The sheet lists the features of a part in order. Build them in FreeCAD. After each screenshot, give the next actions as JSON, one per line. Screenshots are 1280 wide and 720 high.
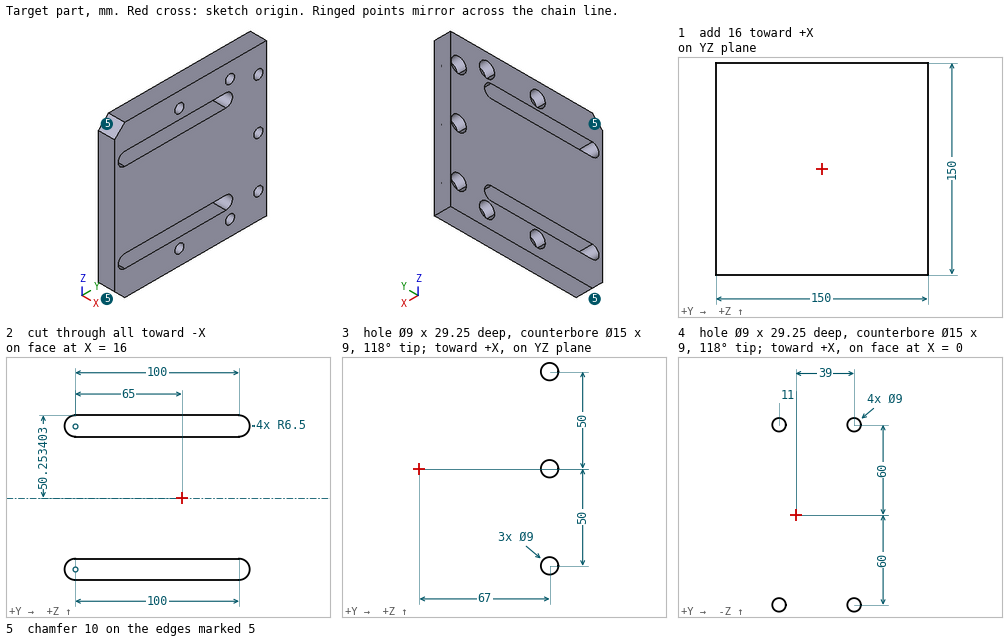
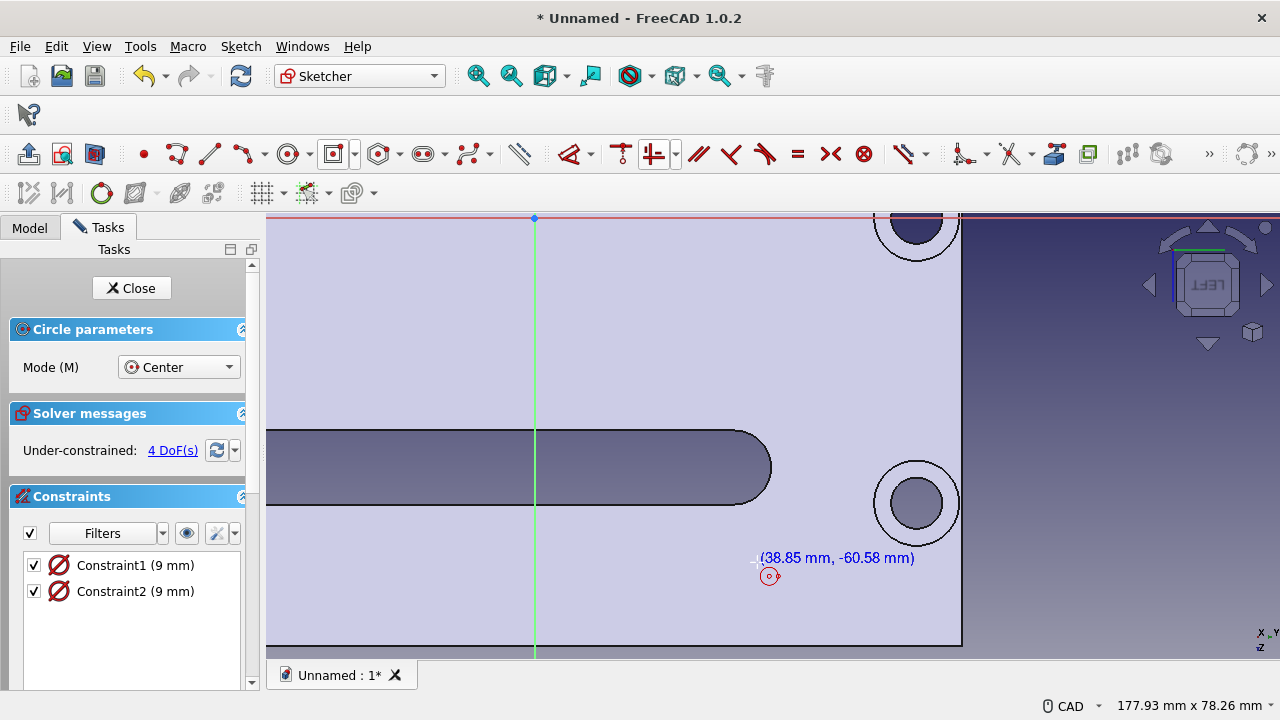
{"action": "left_click", "coordinate": [757, 560]}
{"action": "mouse_move", "coordinate": [775, 542]}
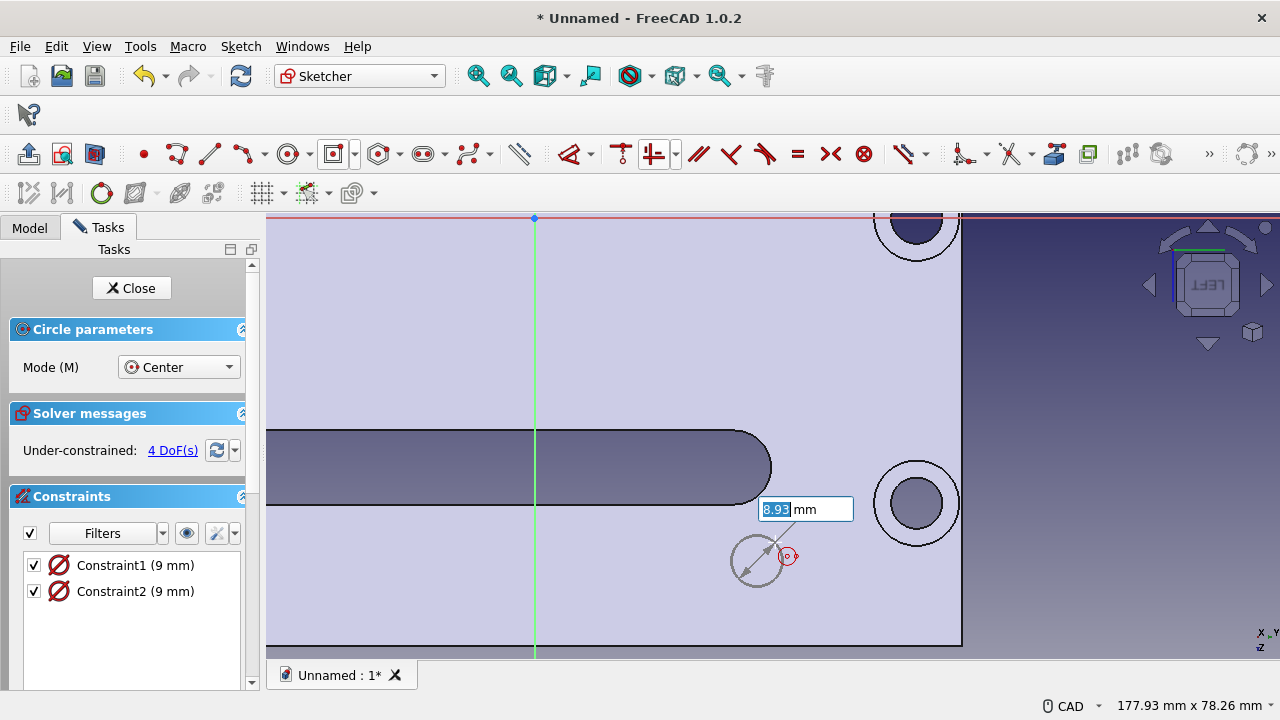
{"action": "type", "text": "9"}
{"action": "key", "text": "Return"}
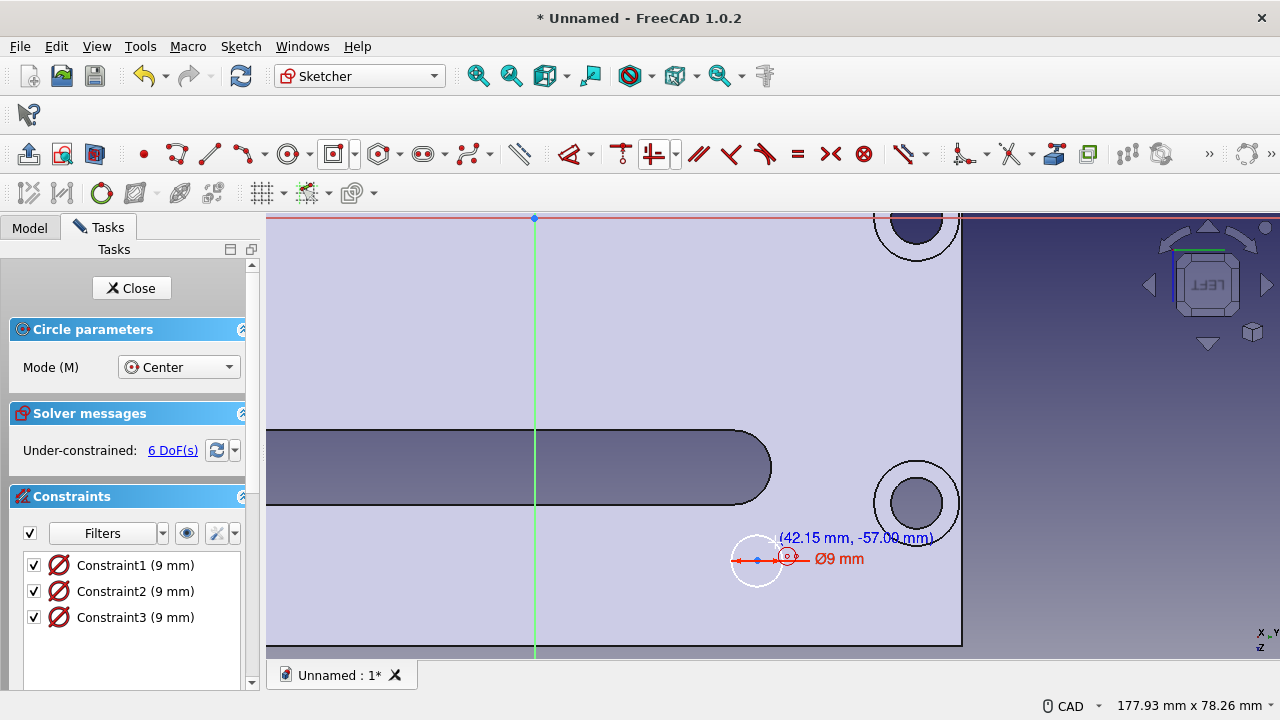
{"action": "left_click", "coordinate": [472, 560]}
{"action": "mouse_move", "coordinate": [490, 542]}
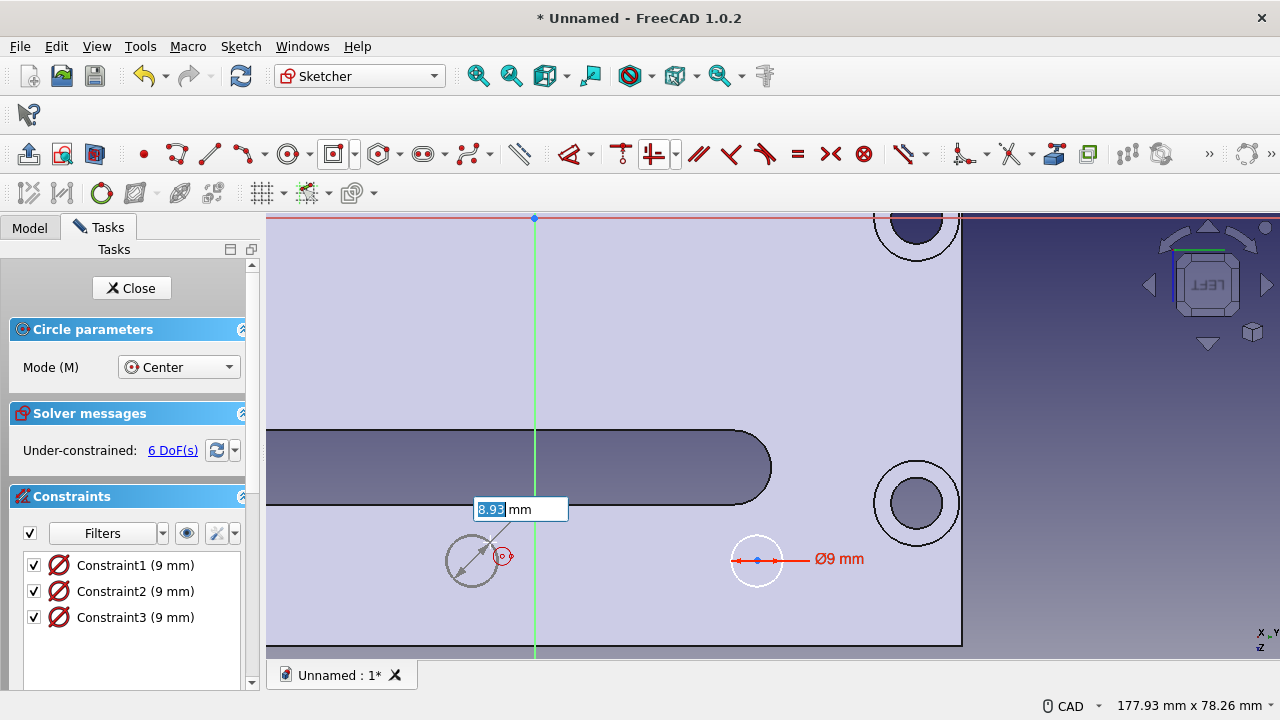
{"action": "type", "text": "9"}
{"action": "key", "text": "Return"}
{"action": "key", "text": "Escape"}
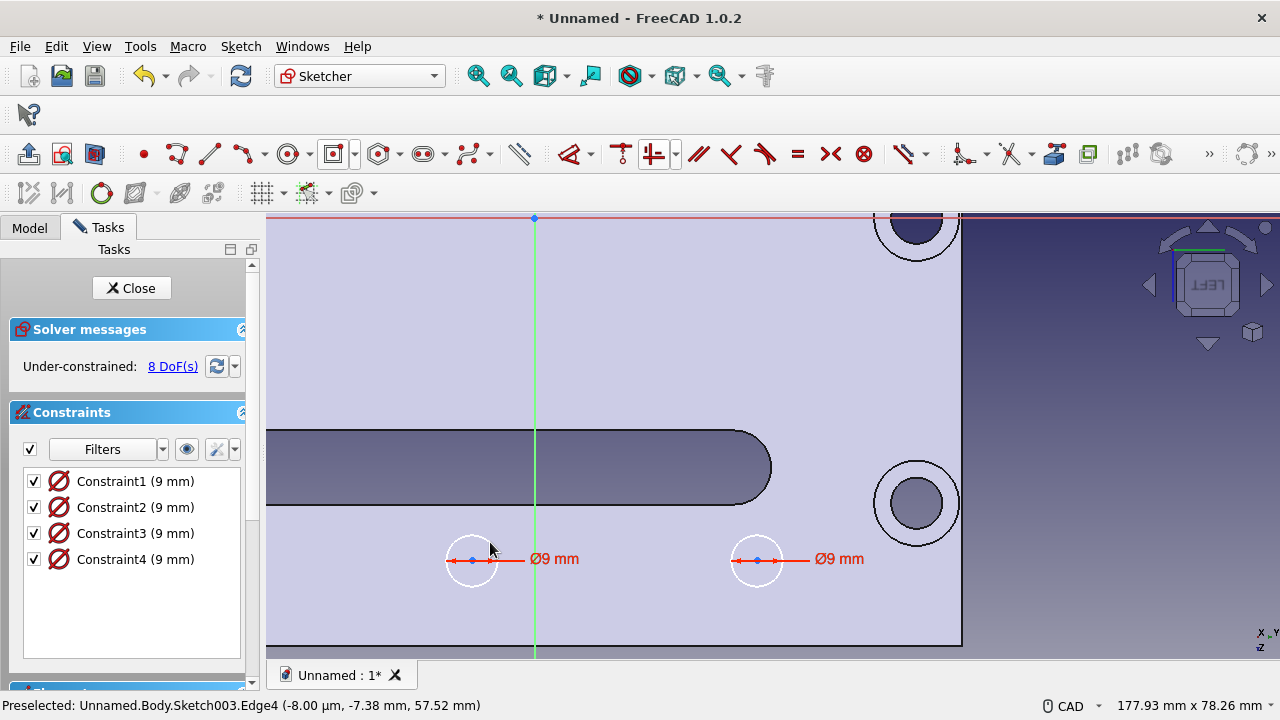
{"action": "scroll", "coordinate": [757, 563], "scroll_direction": "down", "scroll_amount": 5}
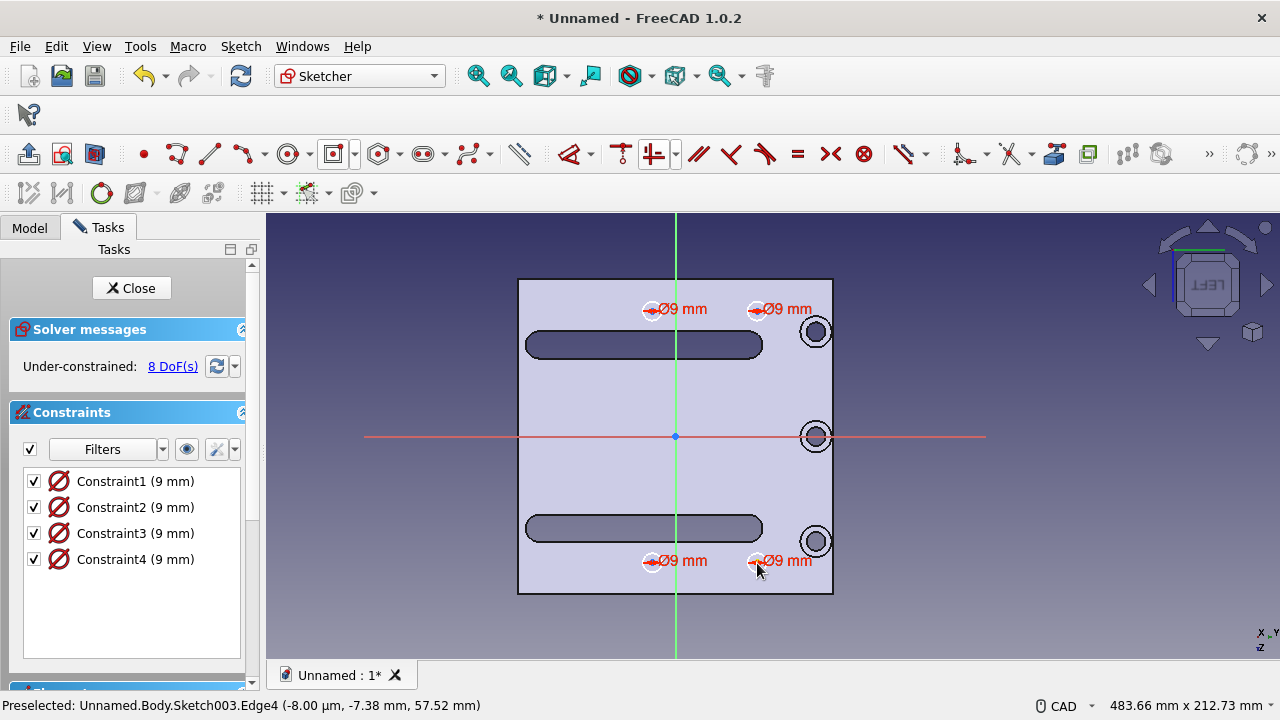
{"action": "left_click", "coordinate": [757, 311]}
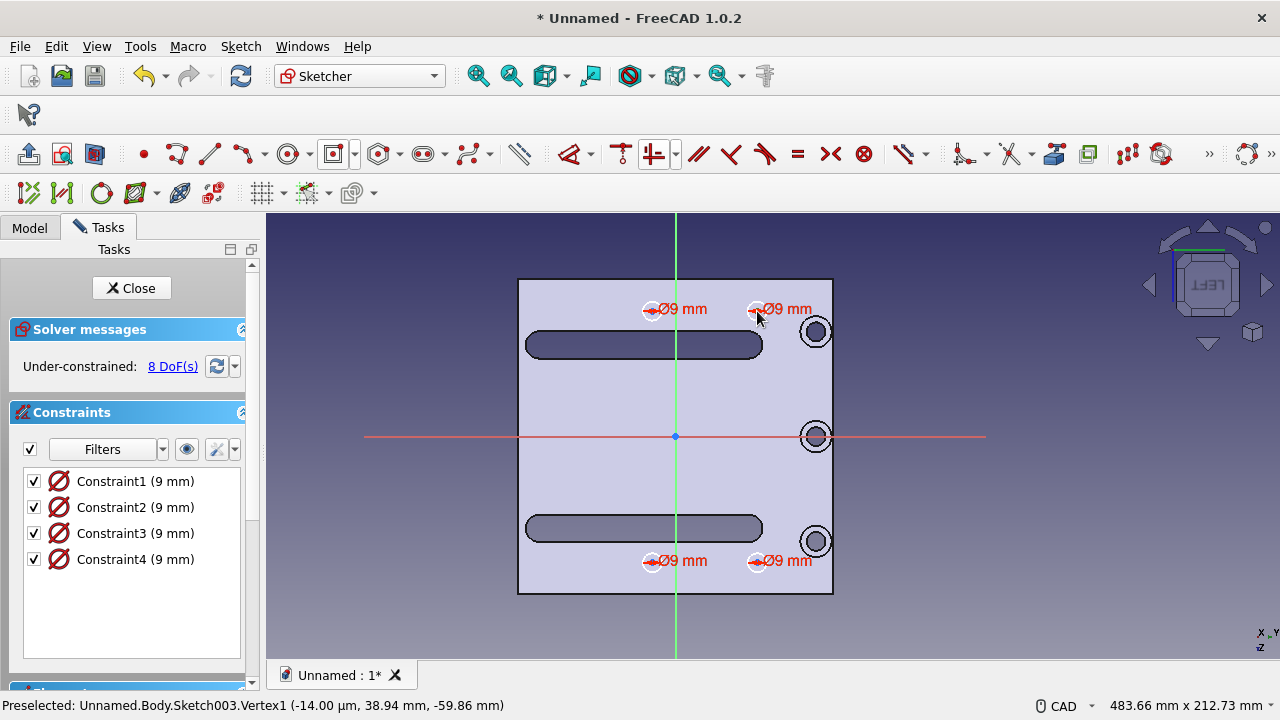
{"action": "left_click", "coordinate": [652, 311]}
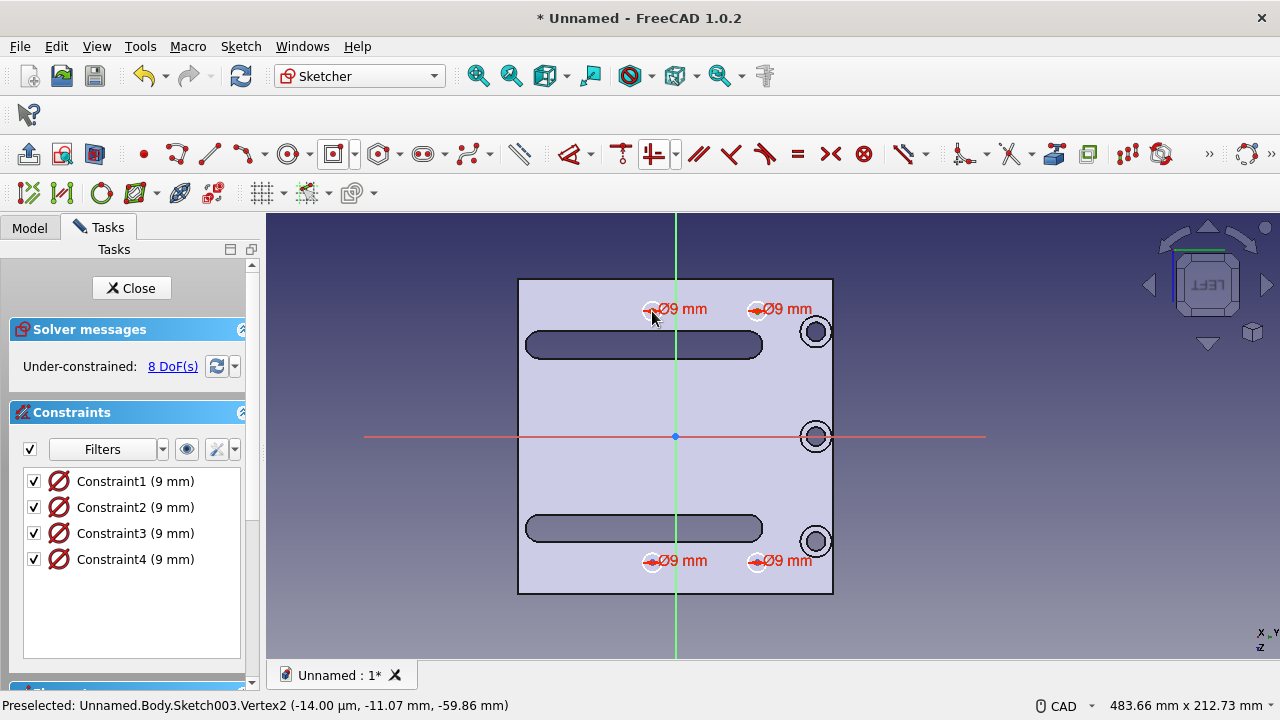
{"action": "left_click", "coordinate": [676, 154]}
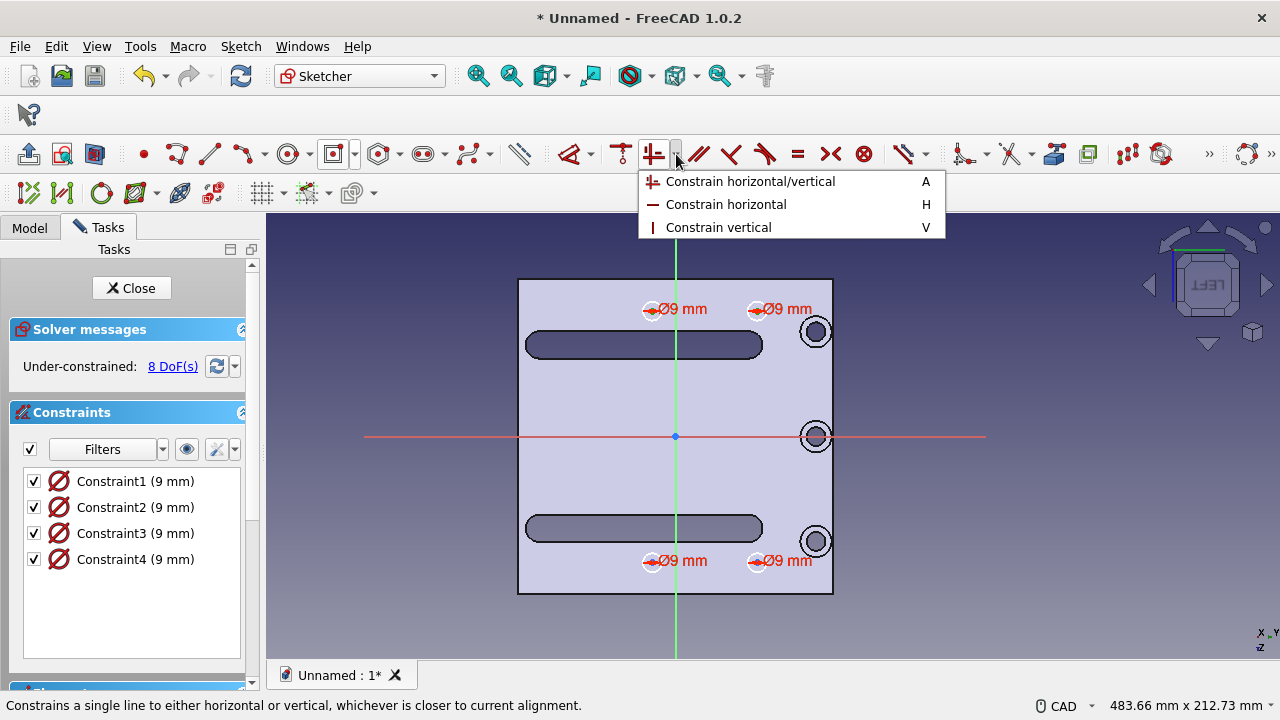
{"action": "left_click", "coordinate": [792, 204]}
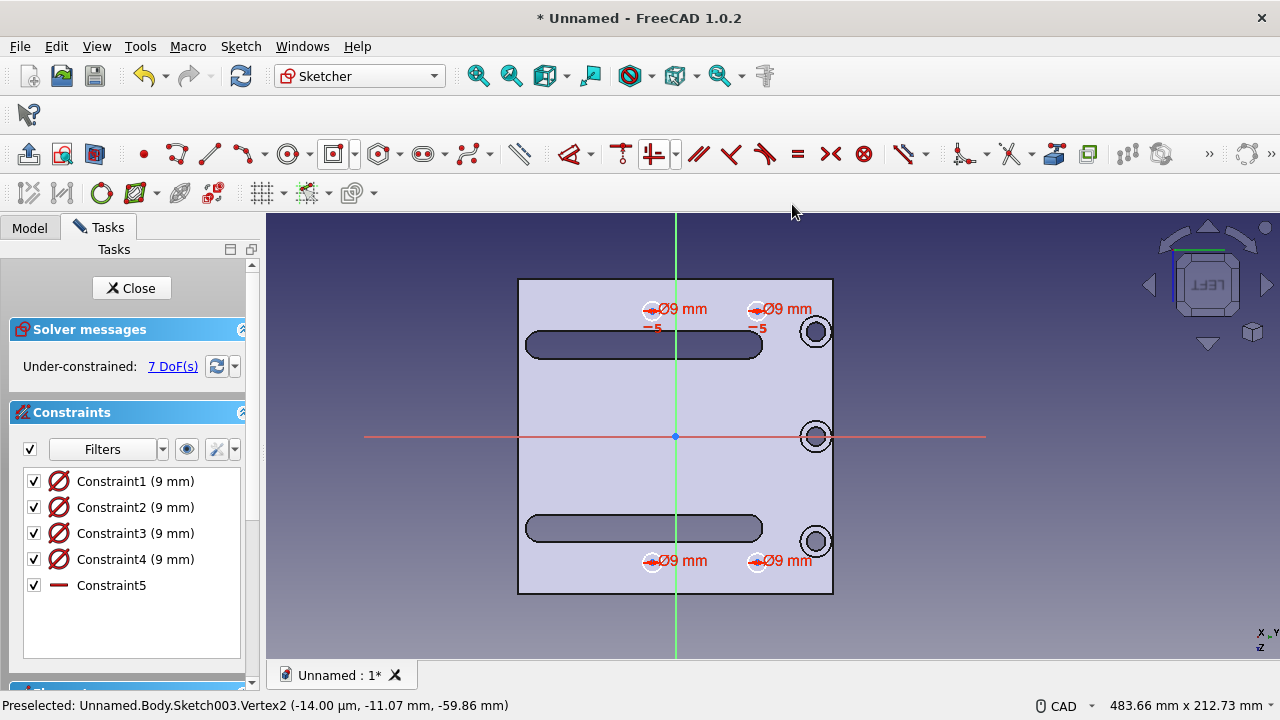
{"action": "left_click", "coordinate": [757, 311]}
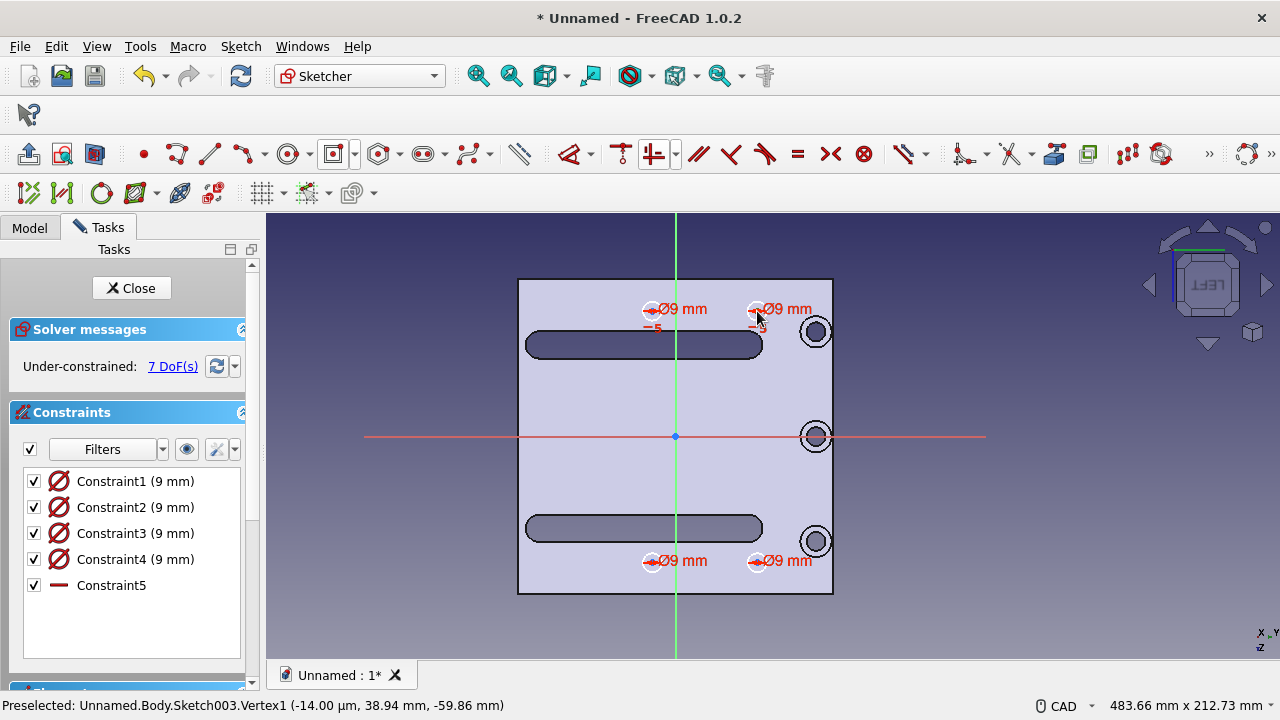
{"action": "left_click", "coordinate": [757, 563]}